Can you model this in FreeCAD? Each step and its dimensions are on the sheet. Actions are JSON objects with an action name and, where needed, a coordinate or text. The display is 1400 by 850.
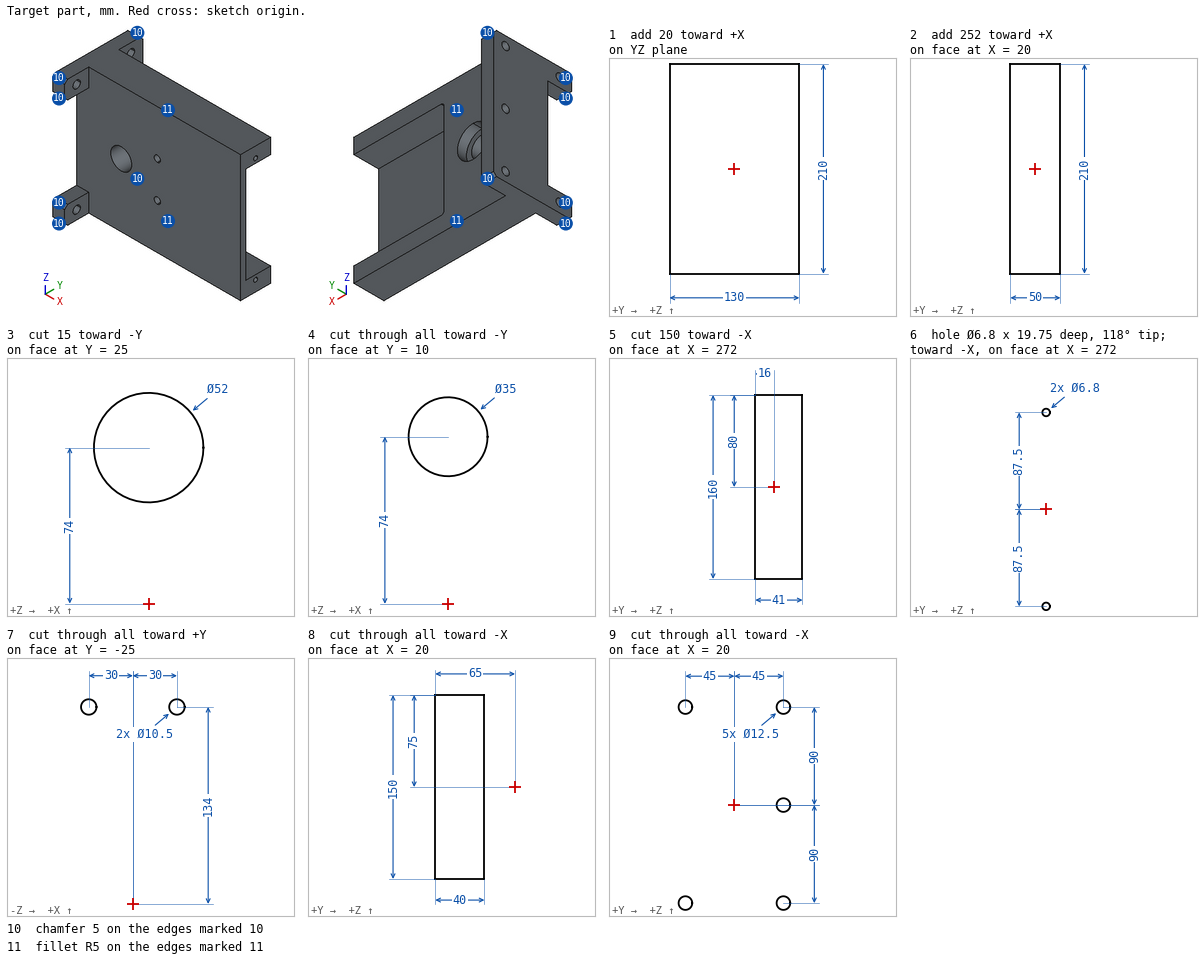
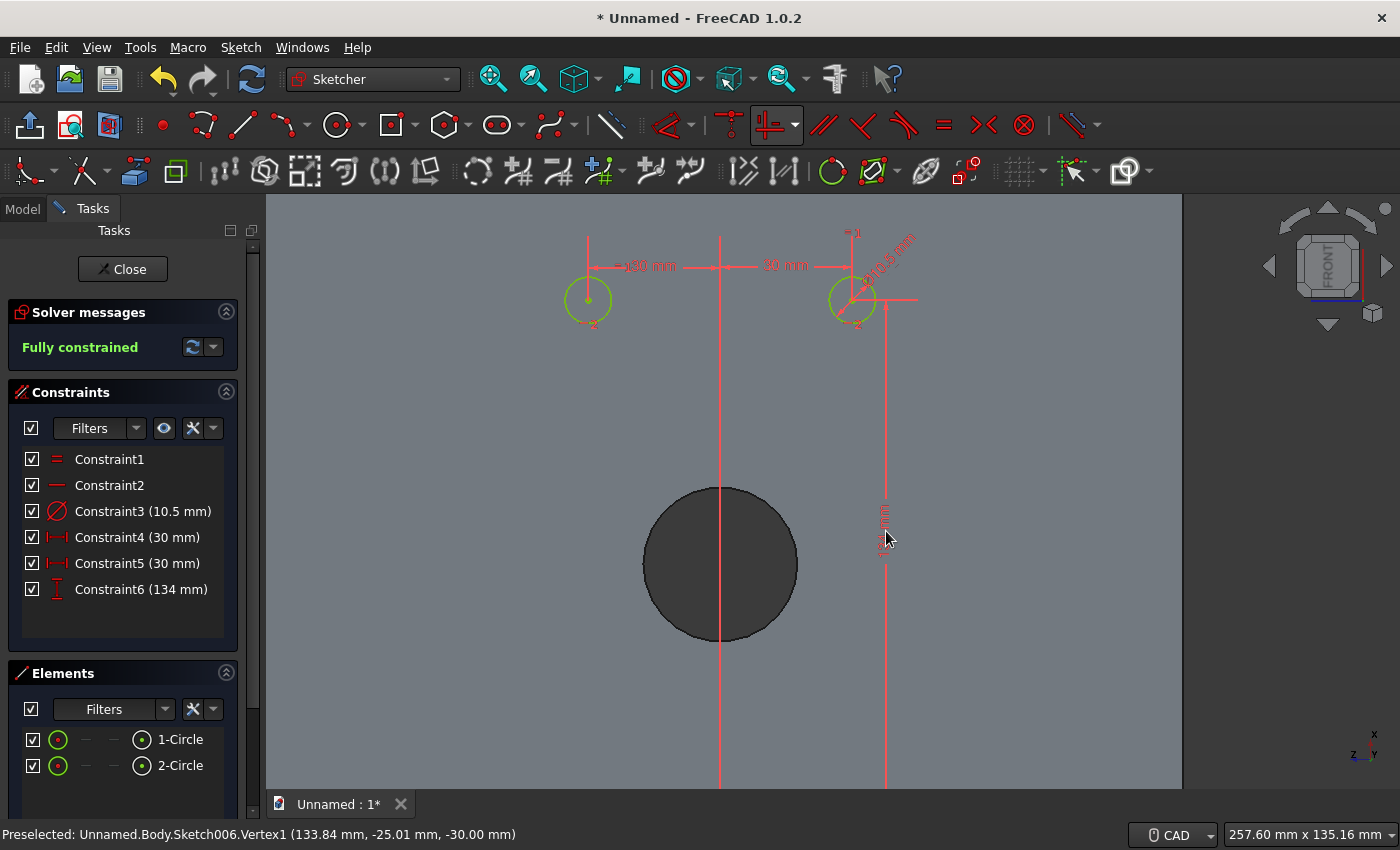
{"action": "left_click", "coordinate": [123, 269]}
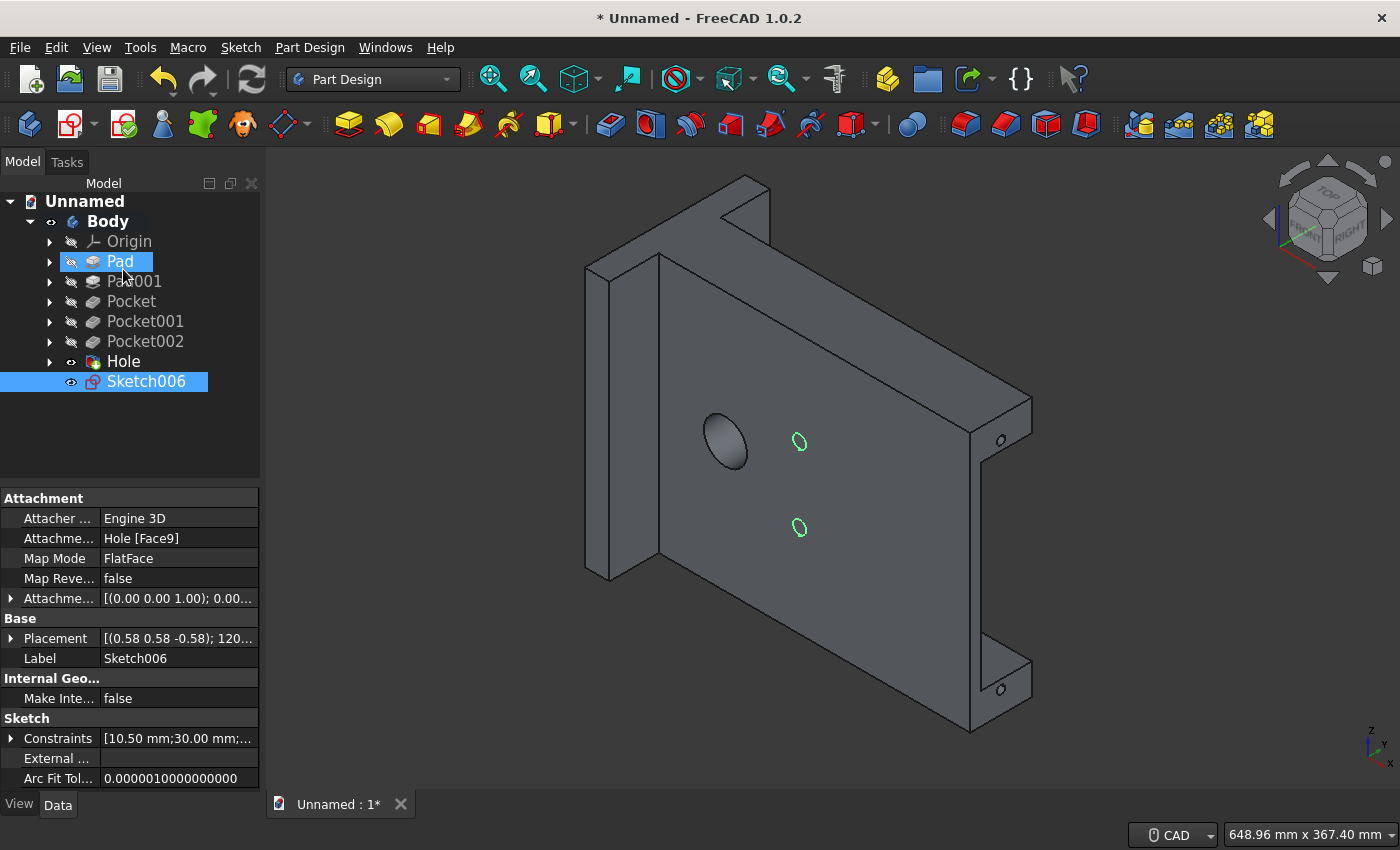
{"action": "left_click", "coordinate": [612, 124]}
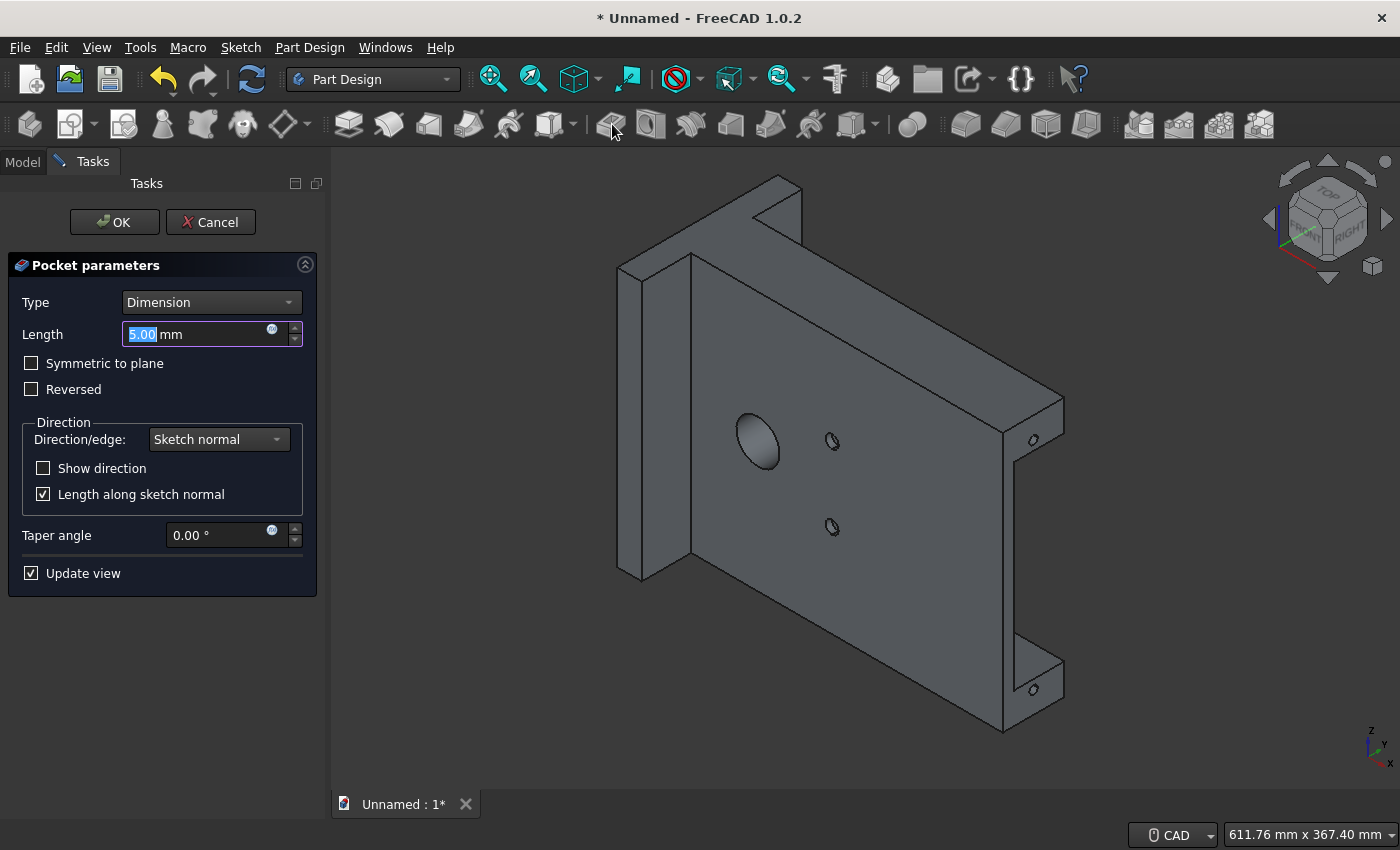
{"action": "left_click", "coordinate": [212, 302]}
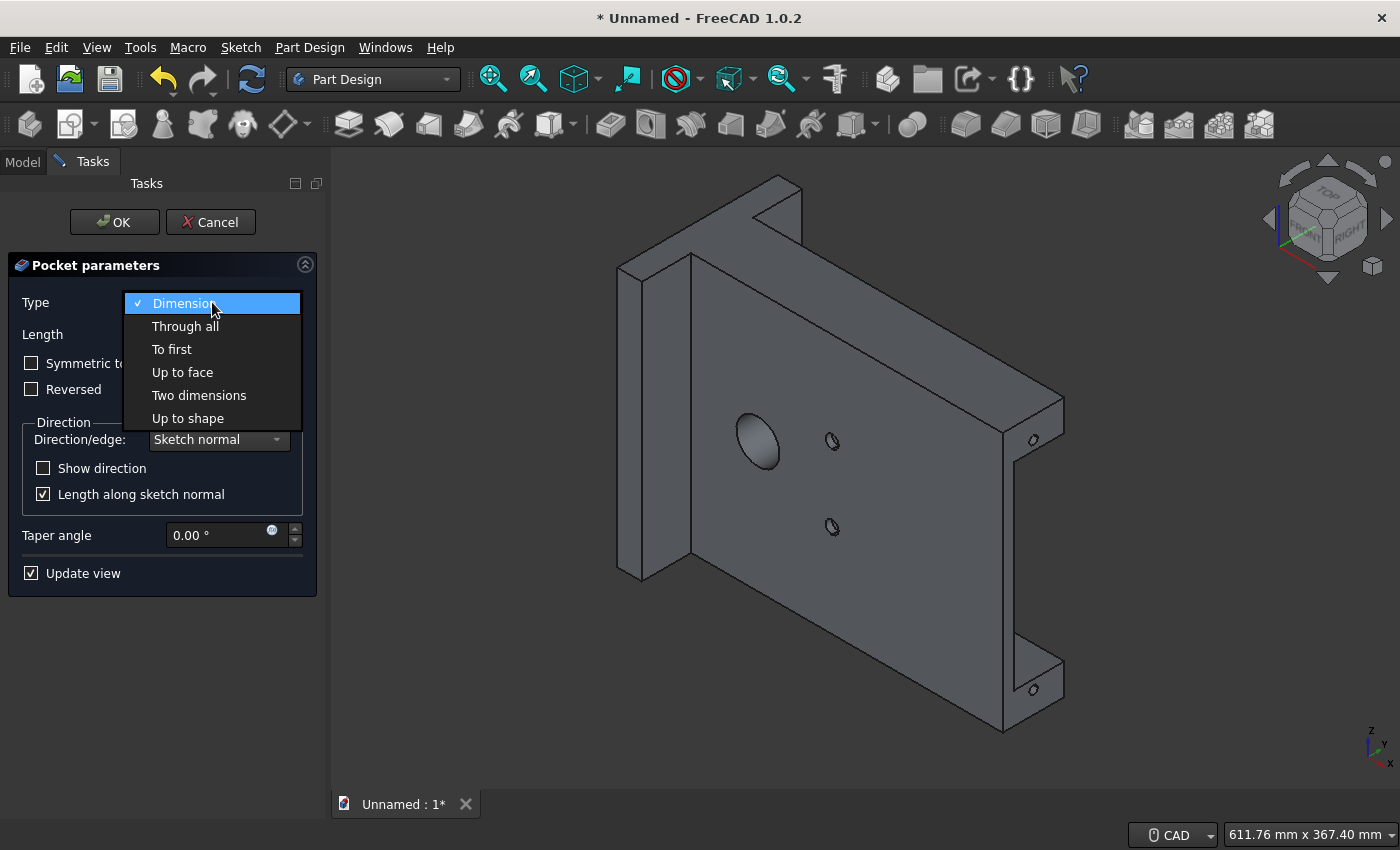
{"action": "left_click", "coordinate": [212, 326]}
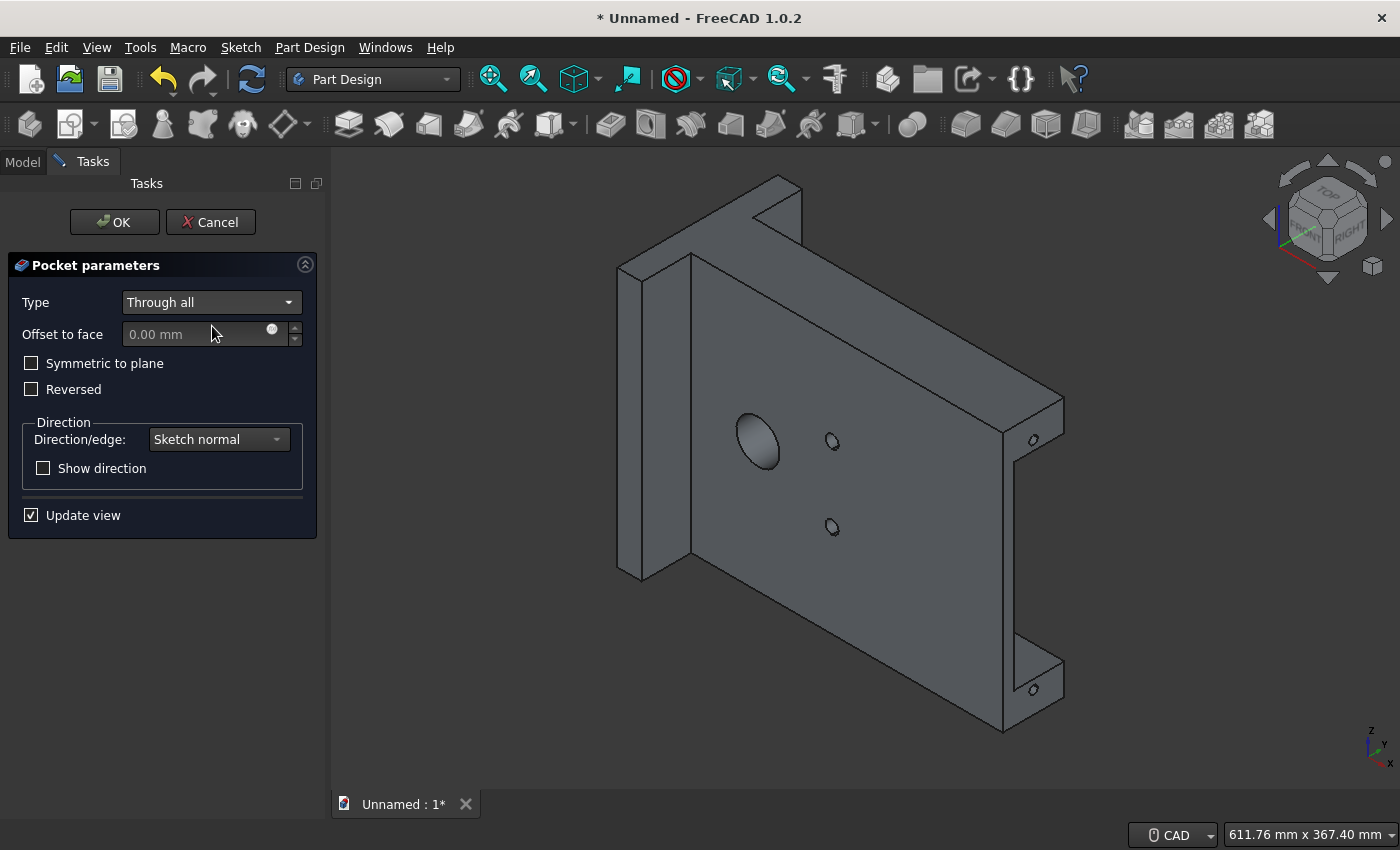
{"action": "left_click", "coordinate": [115, 222]}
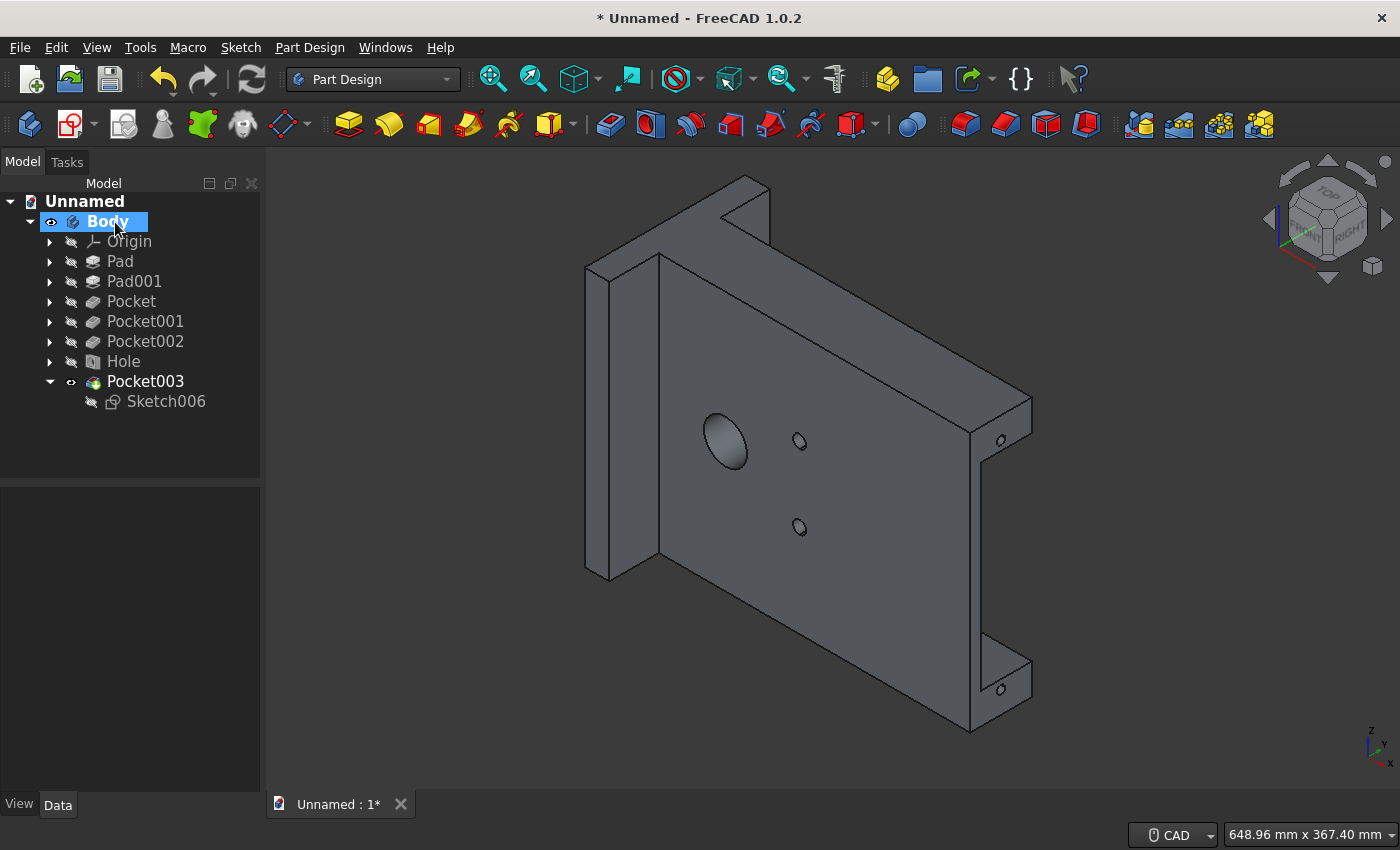
{"action": "left_click", "coordinate": [634, 502]}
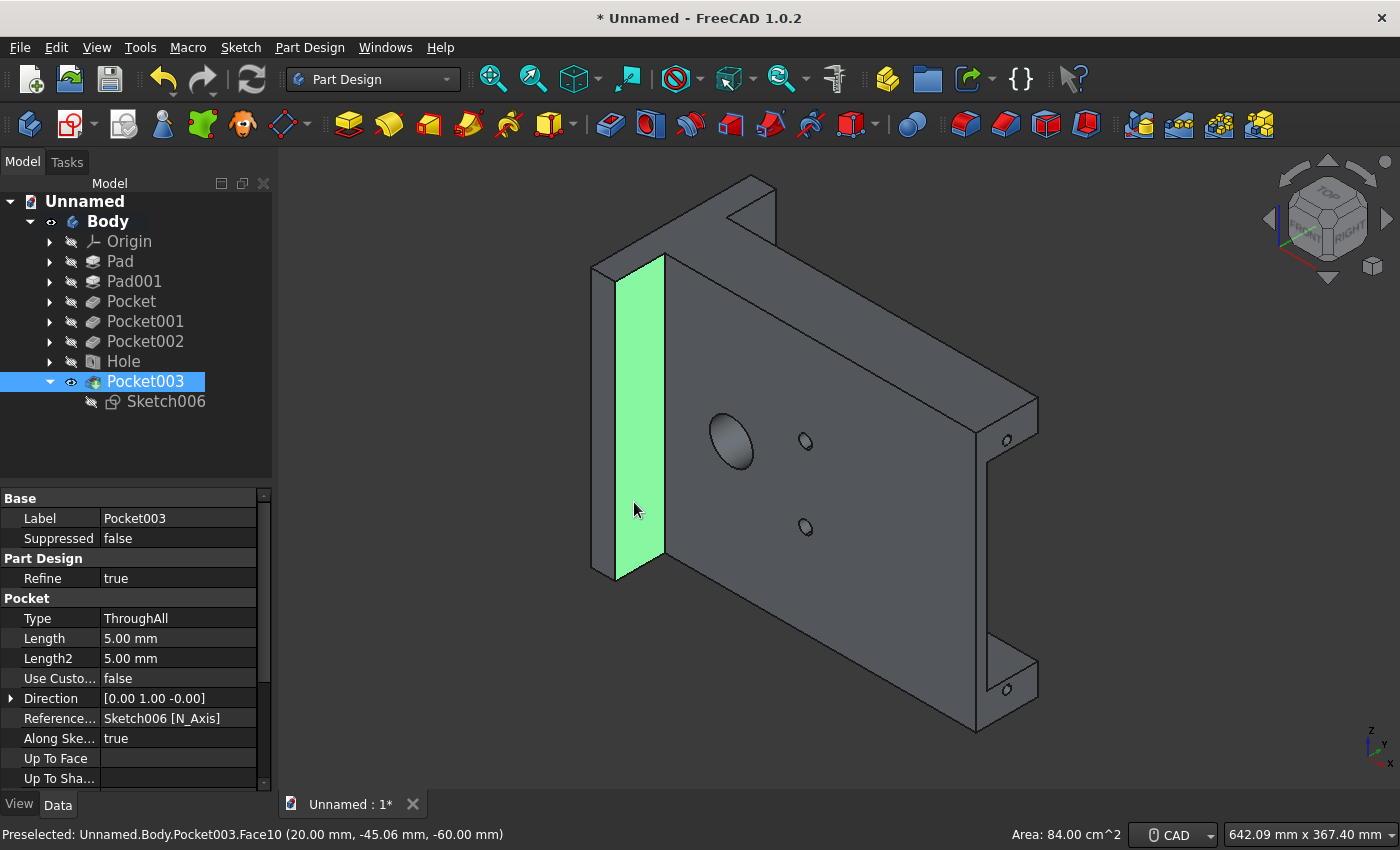
{"action": "left_click", "coordinate": [70, 124]}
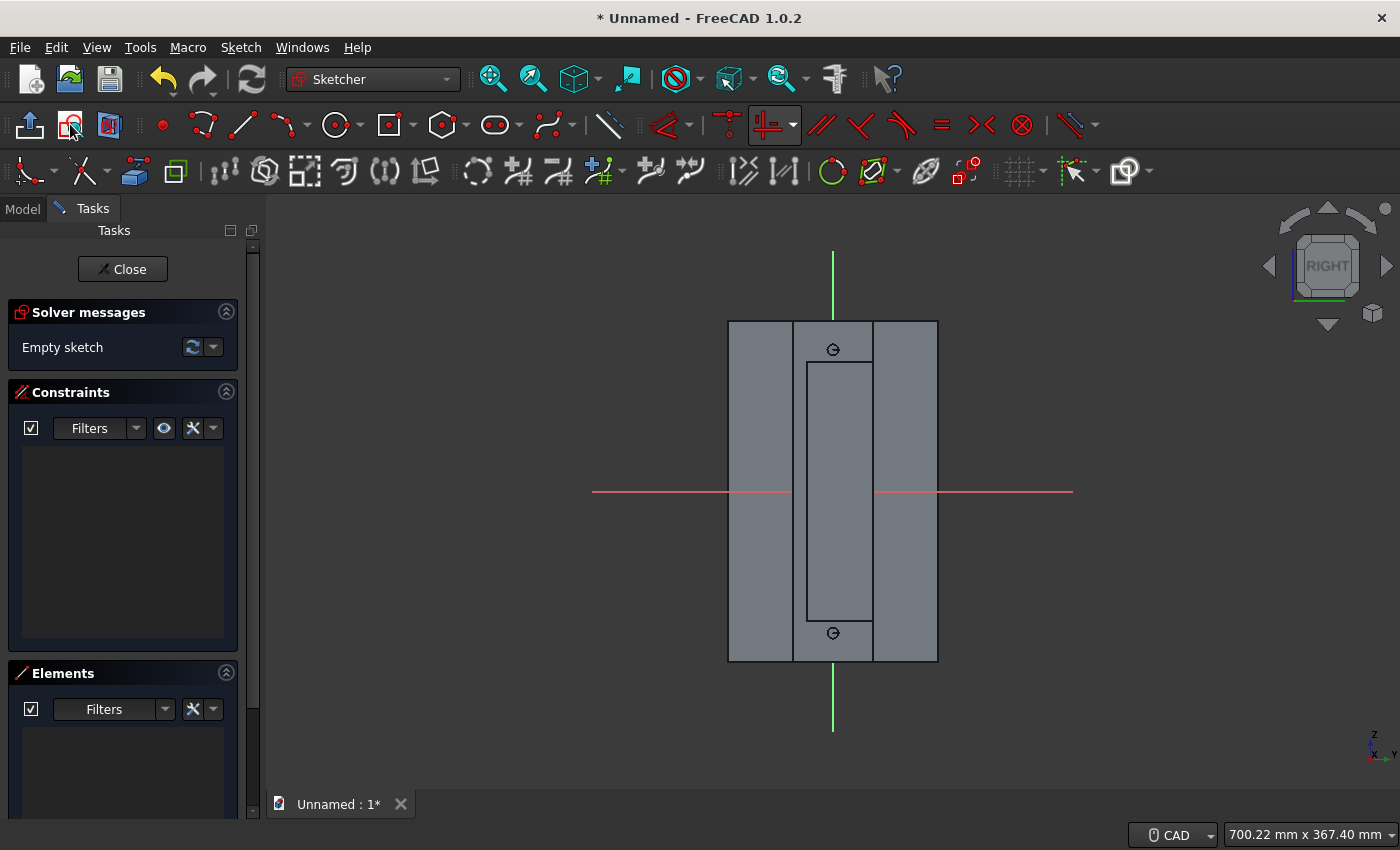
{"action": "left_click", "coordinate": [110, 126]}